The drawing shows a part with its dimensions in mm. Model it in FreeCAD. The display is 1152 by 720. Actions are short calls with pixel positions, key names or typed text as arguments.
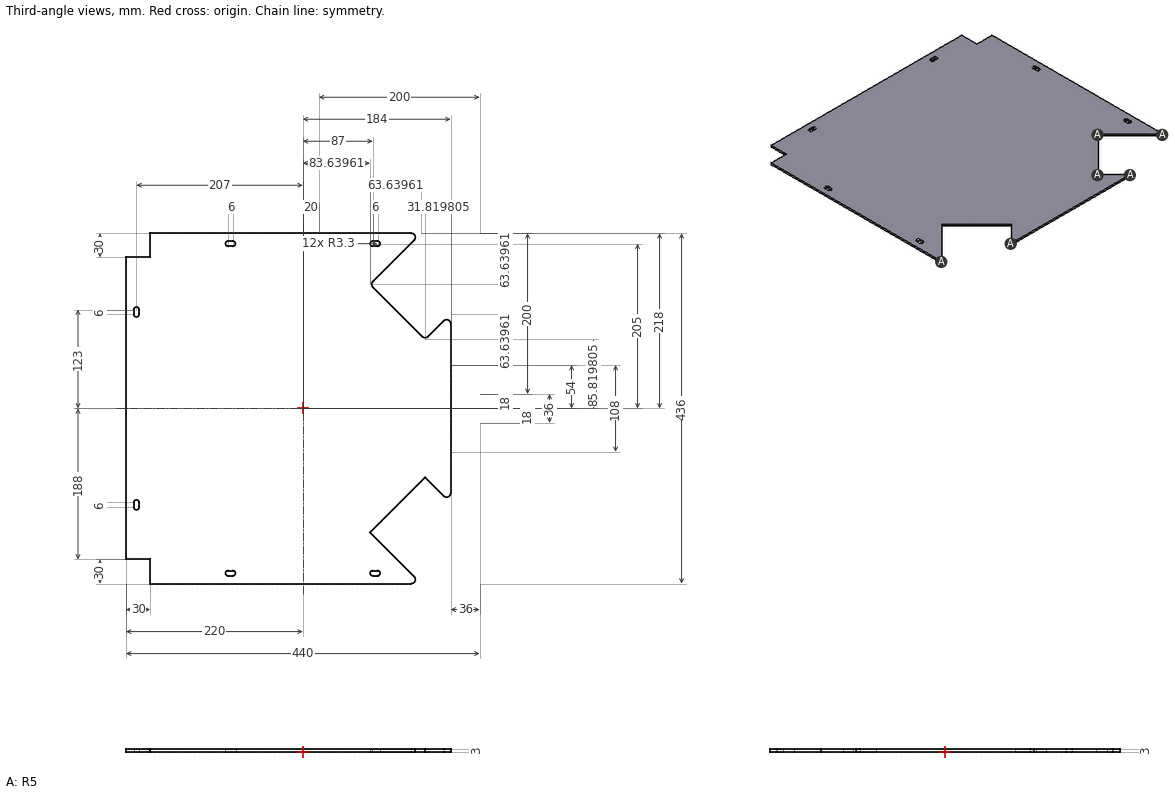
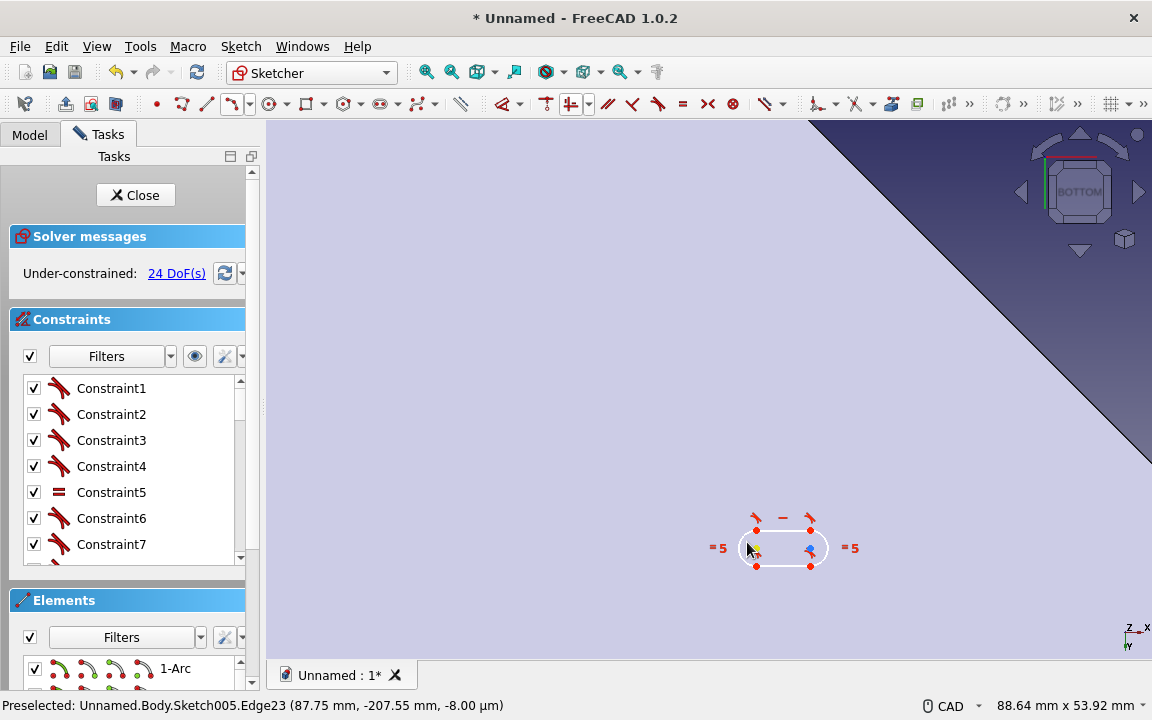
click(742, 538)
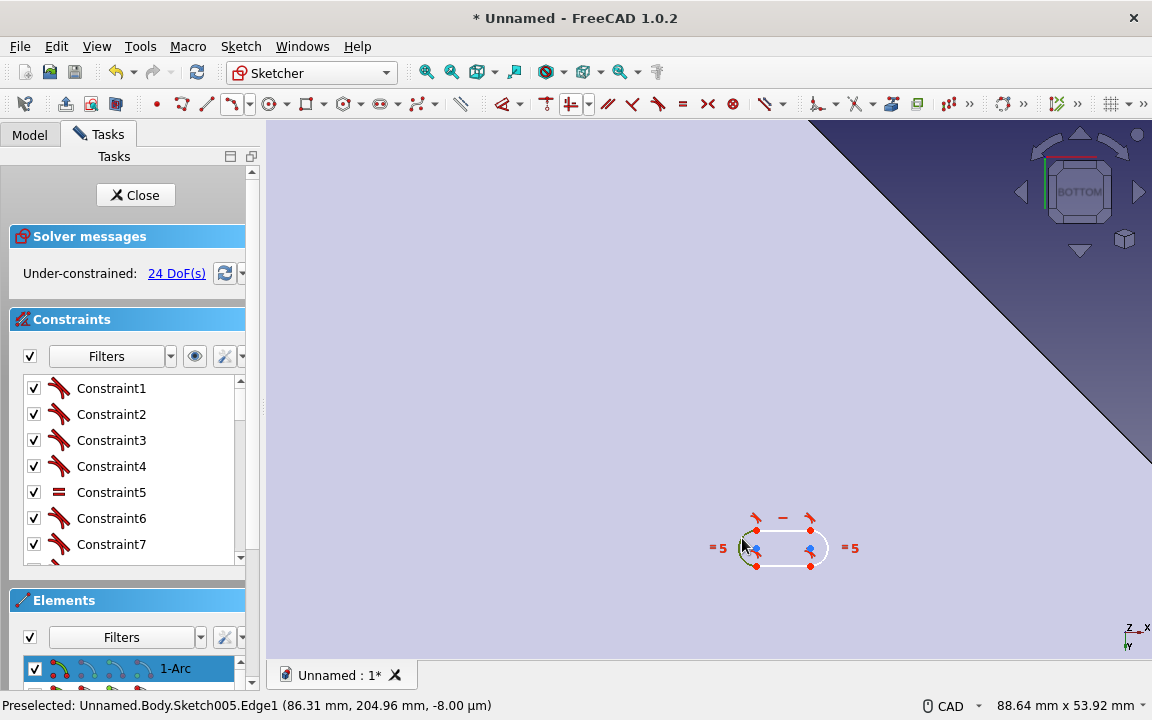
scroll(747, 542, down, 13)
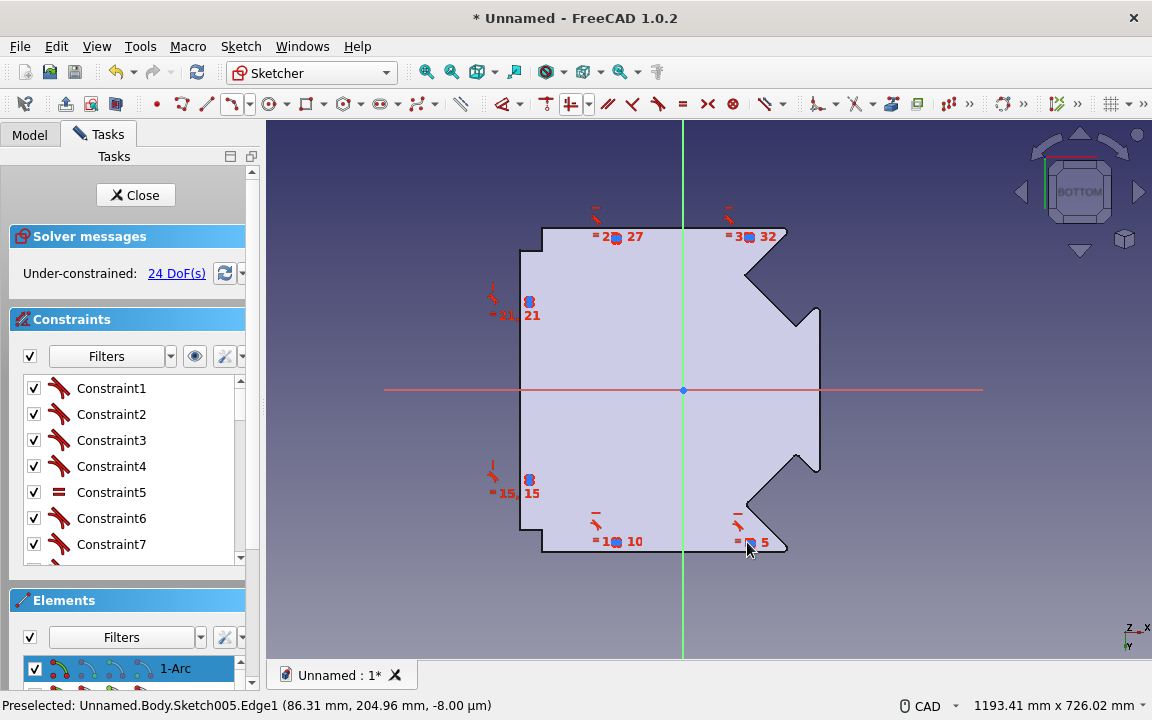
scroll(613, 542, up, 11)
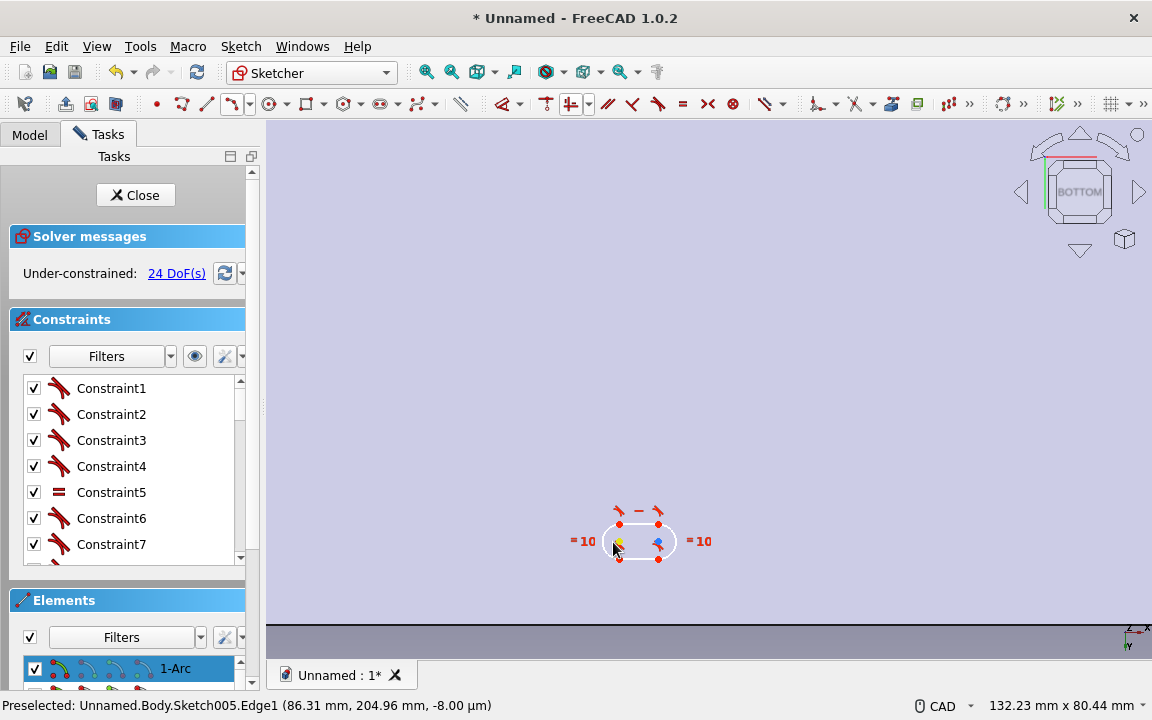
click(606, 532)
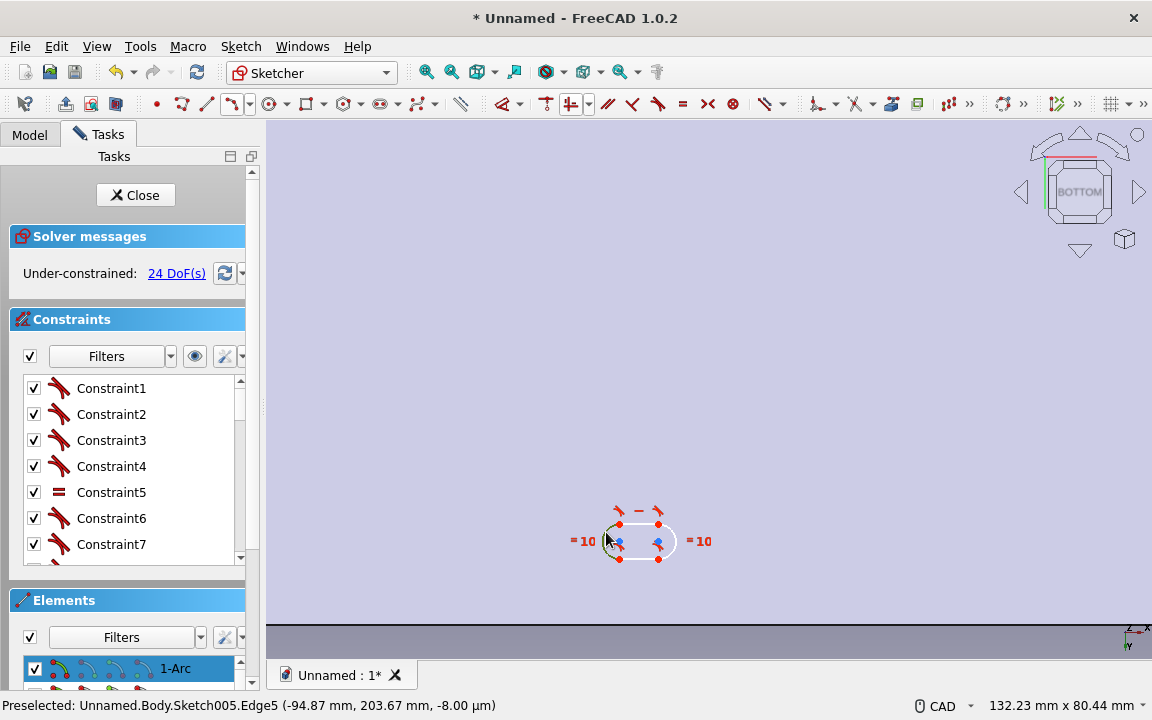
scroll(613, 542, down, 11)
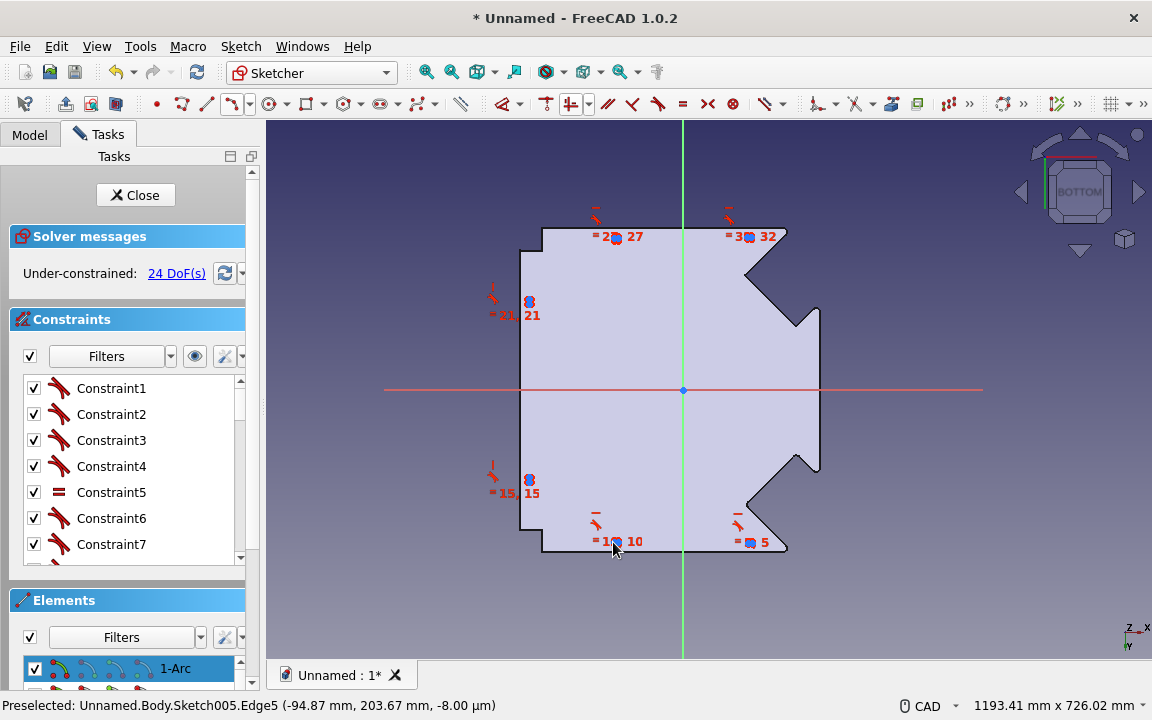
scroll(528, 484, up, 10)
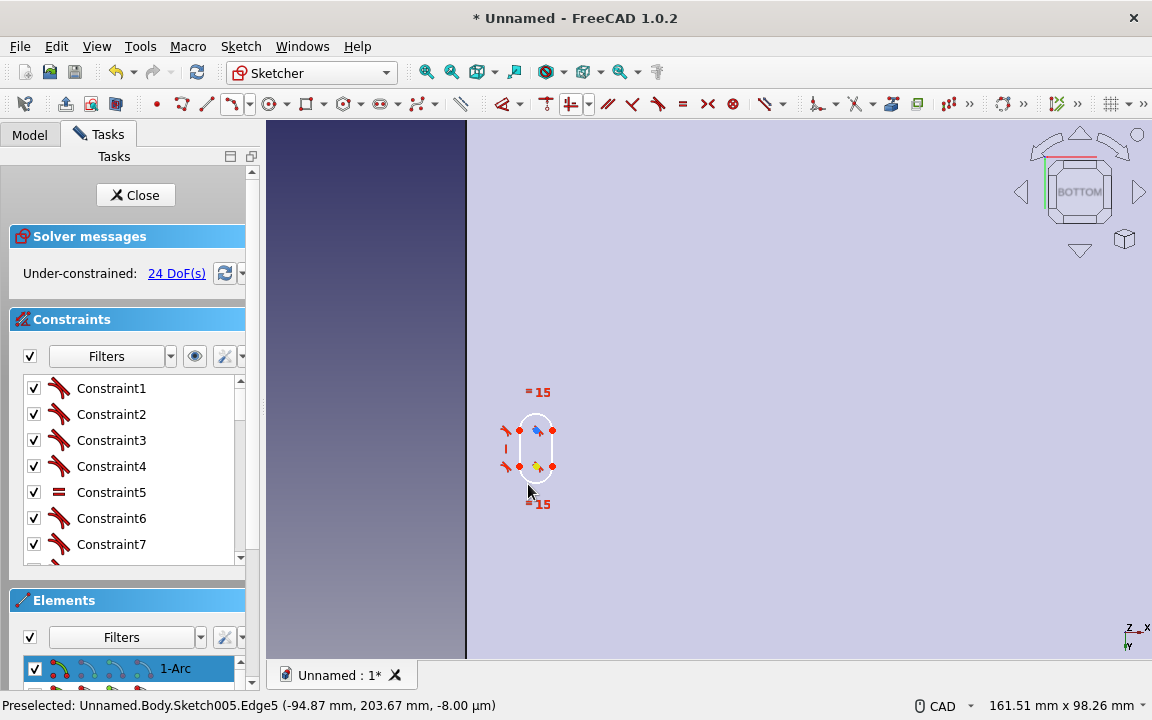
click(527, 480)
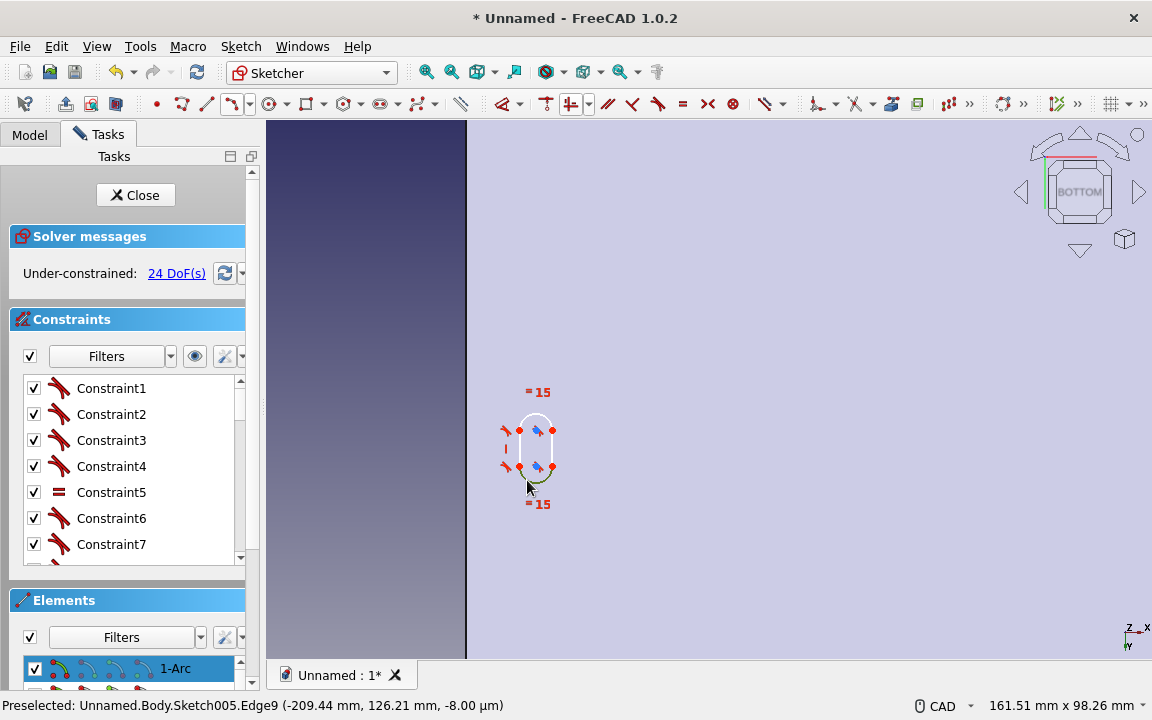
scroll(528, 484, down, 10)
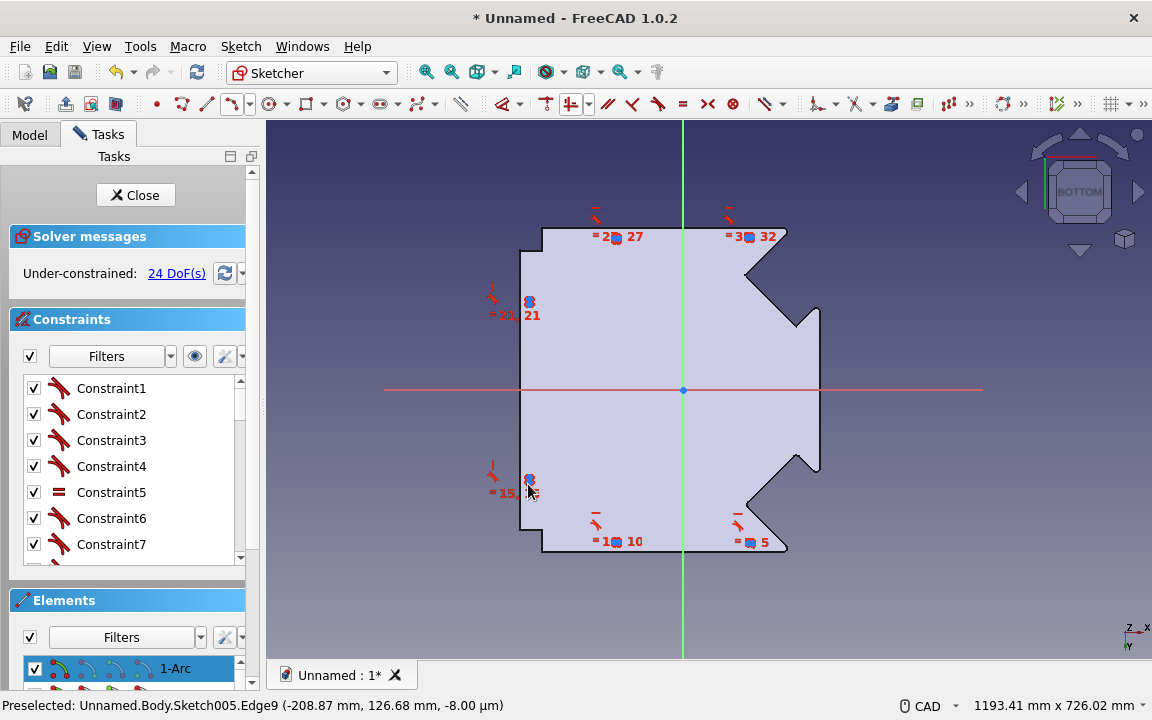
scroll(528, 306, up, 11)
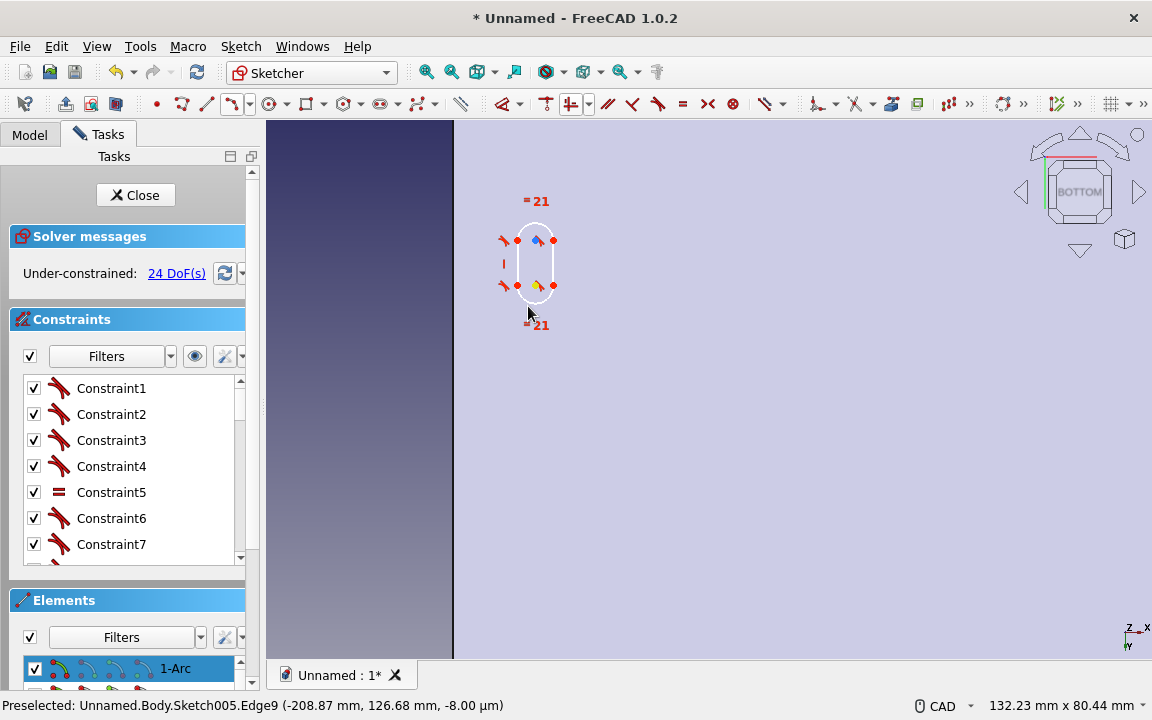
click(525, 300)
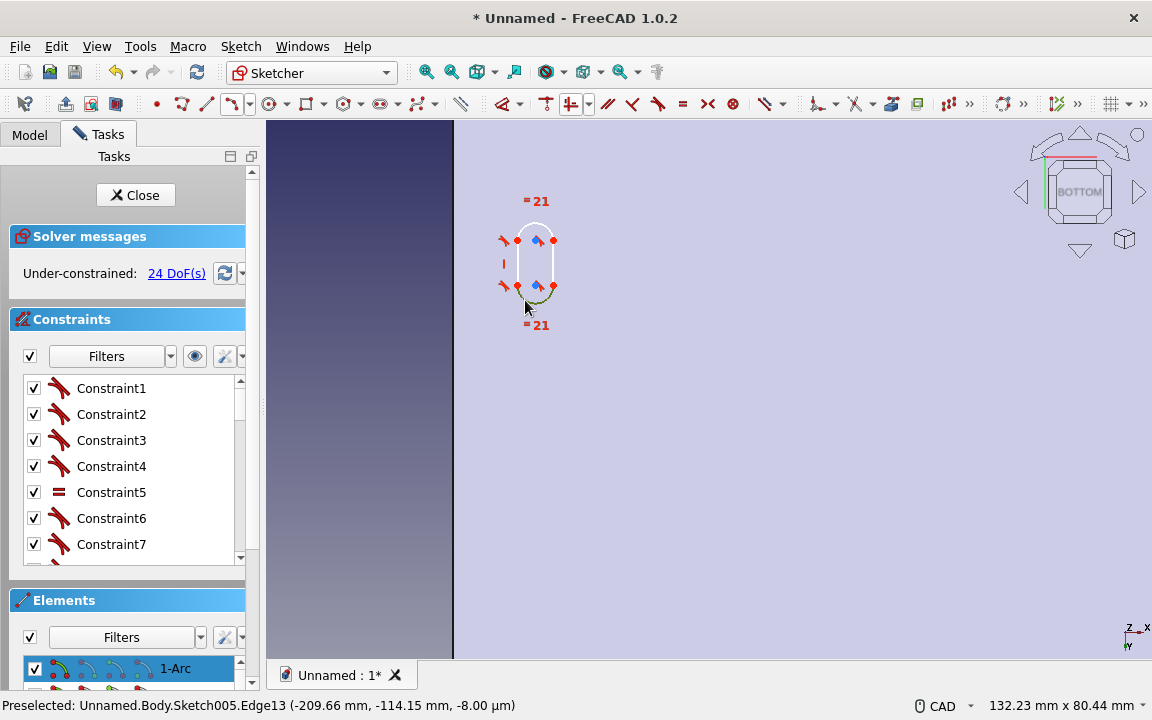
scroll(528, 306, down, 11)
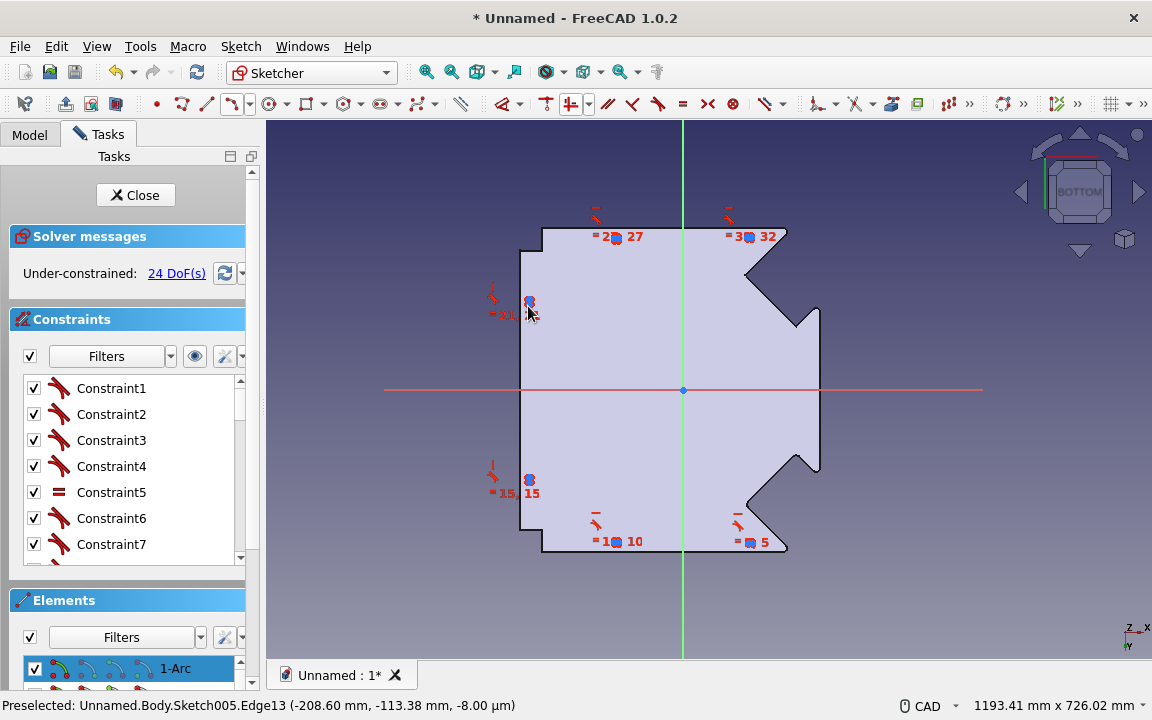
scroll(612, 237, up, 10)